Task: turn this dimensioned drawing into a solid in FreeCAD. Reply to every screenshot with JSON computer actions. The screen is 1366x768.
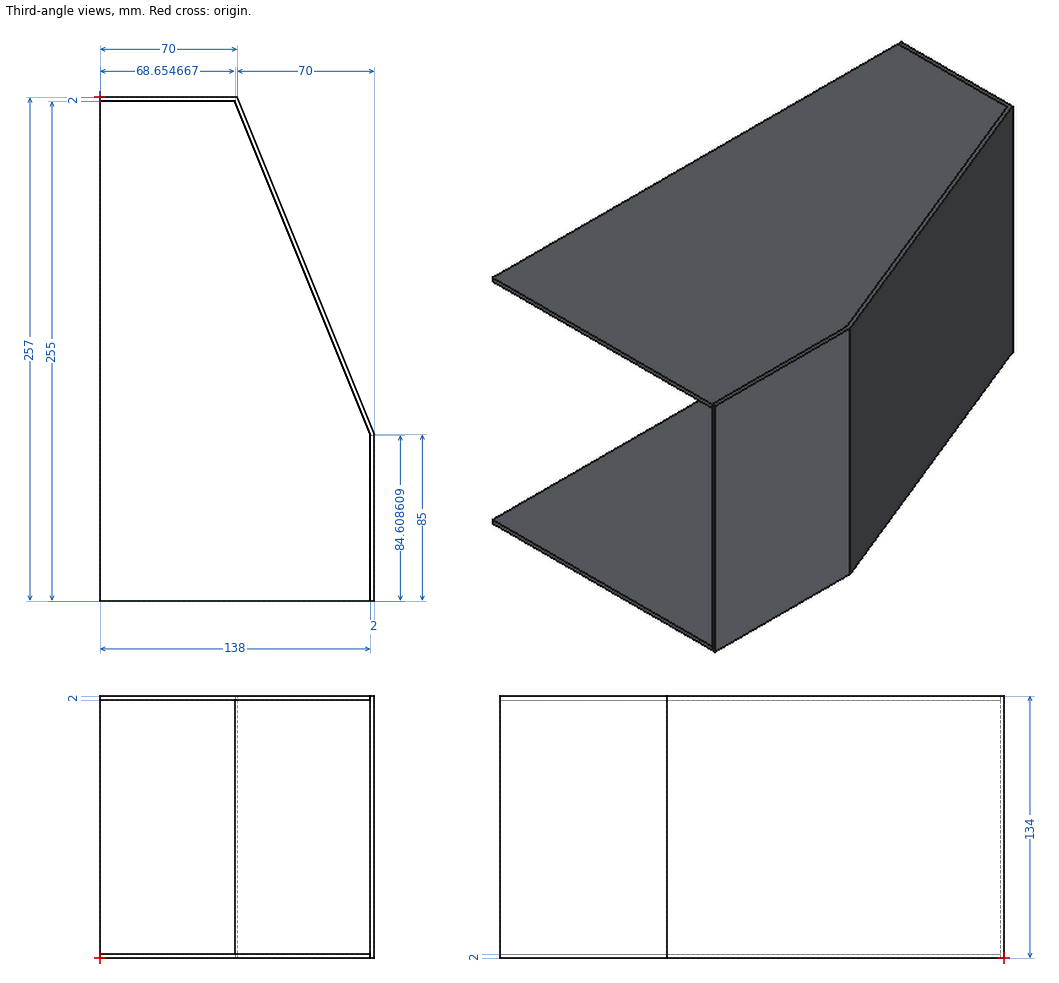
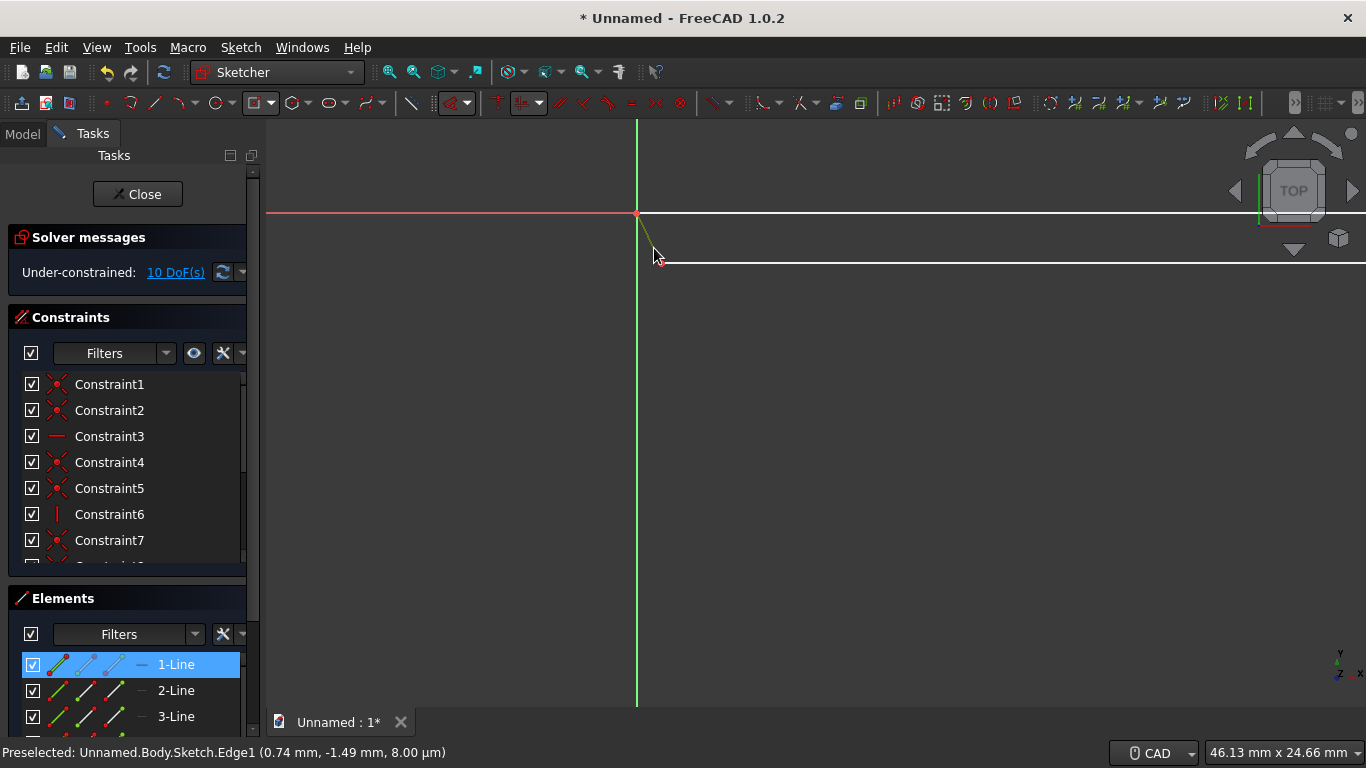
{"action": "key", "text": "v"}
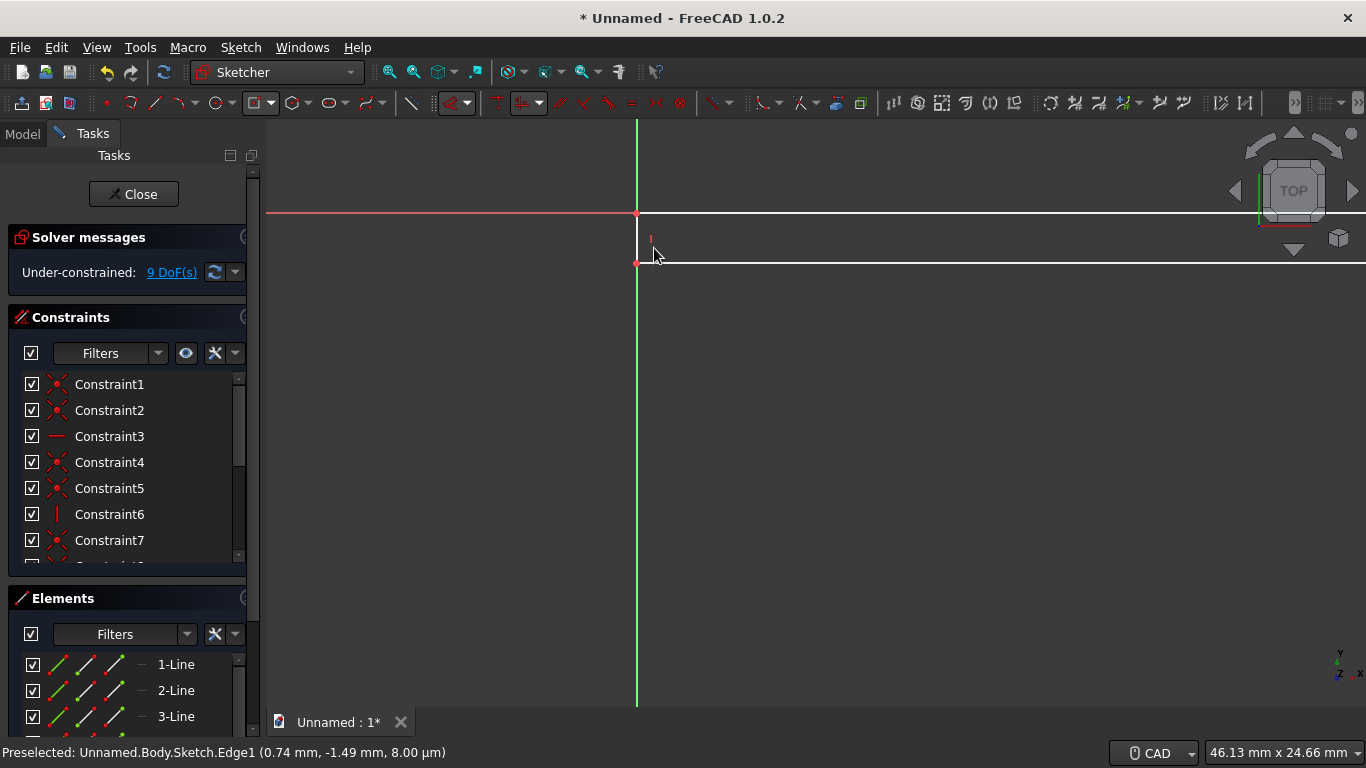
{"action": "scroll", "coordinate": [647, 228], "scroll_direction": "down", "scroll_amount": 14}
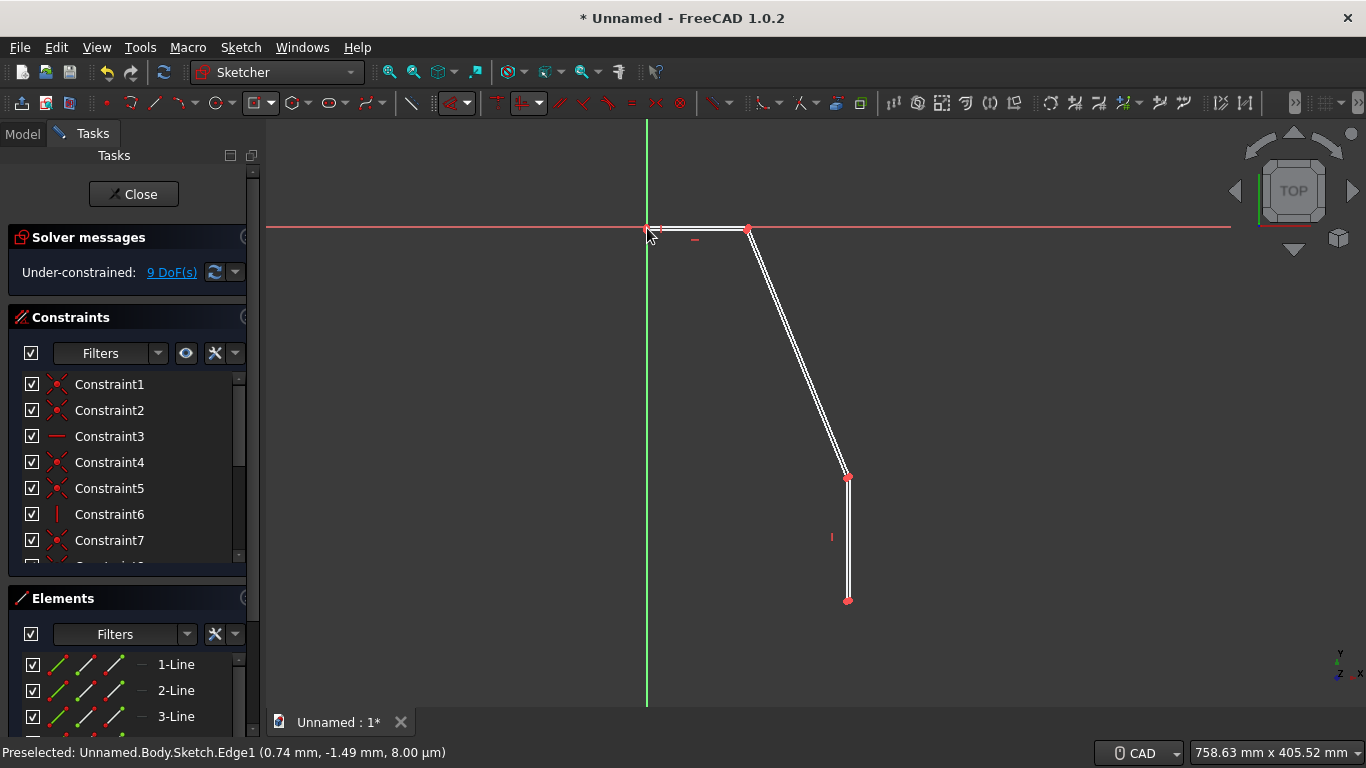
{"action": "scroll", "coordinate": [848, 601], "scroll_direction": "up", "scroll_amount": 14}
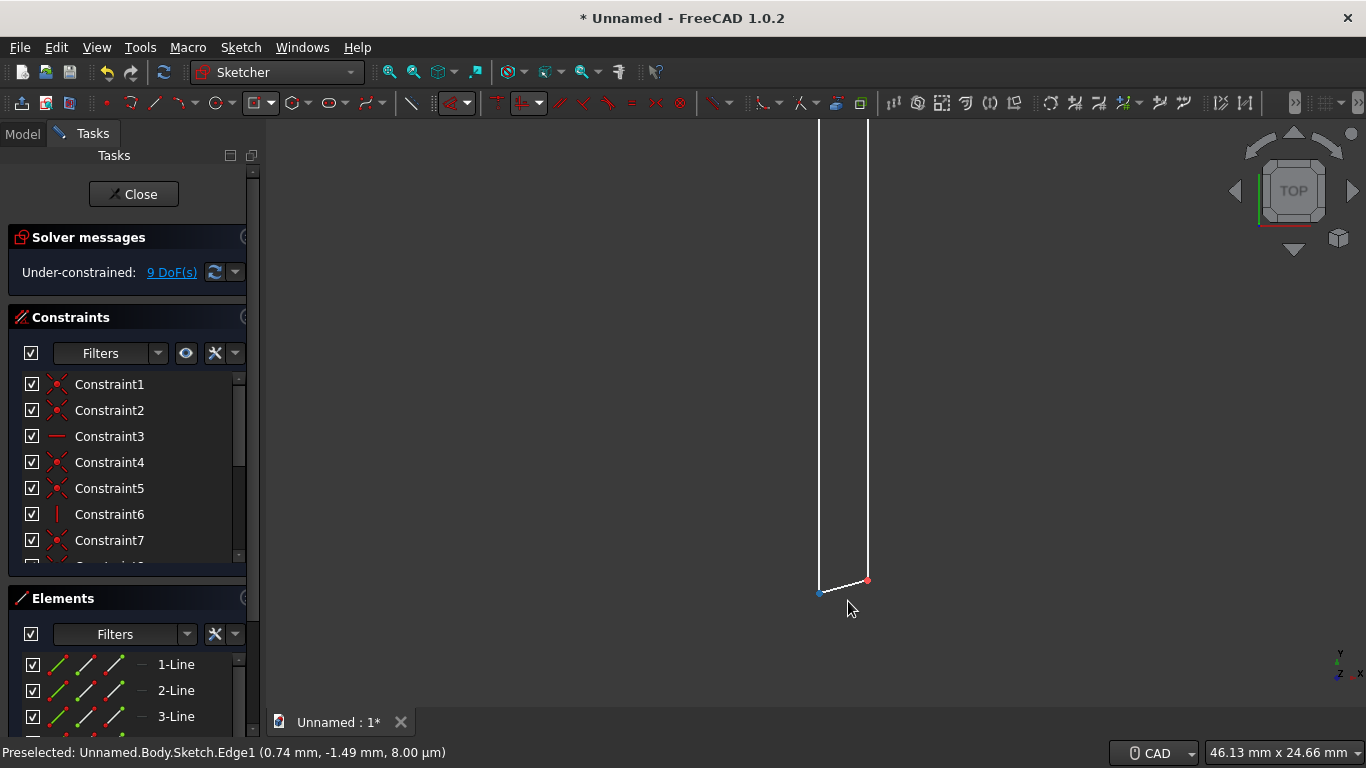
{"action": "left_click", "coordinate": [834, 589]}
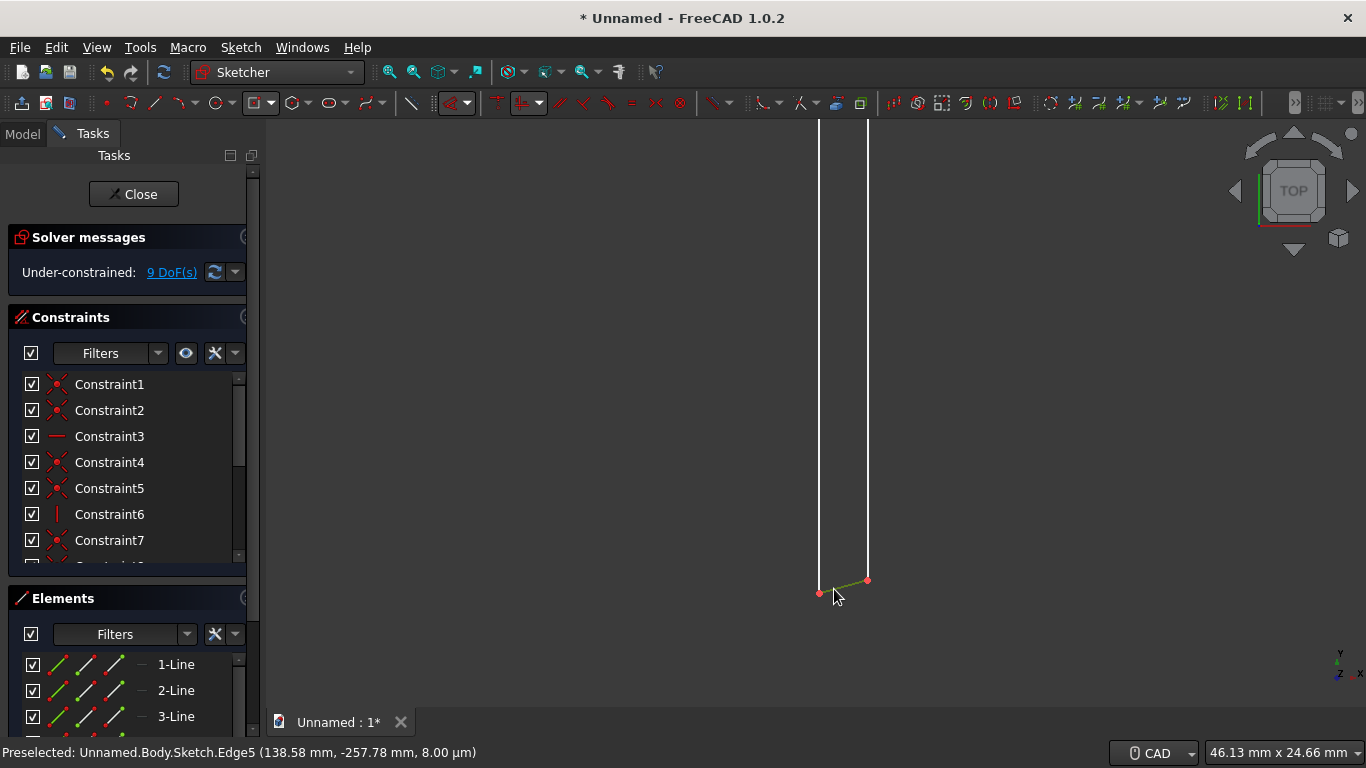
{"action": "key", "text": "h"}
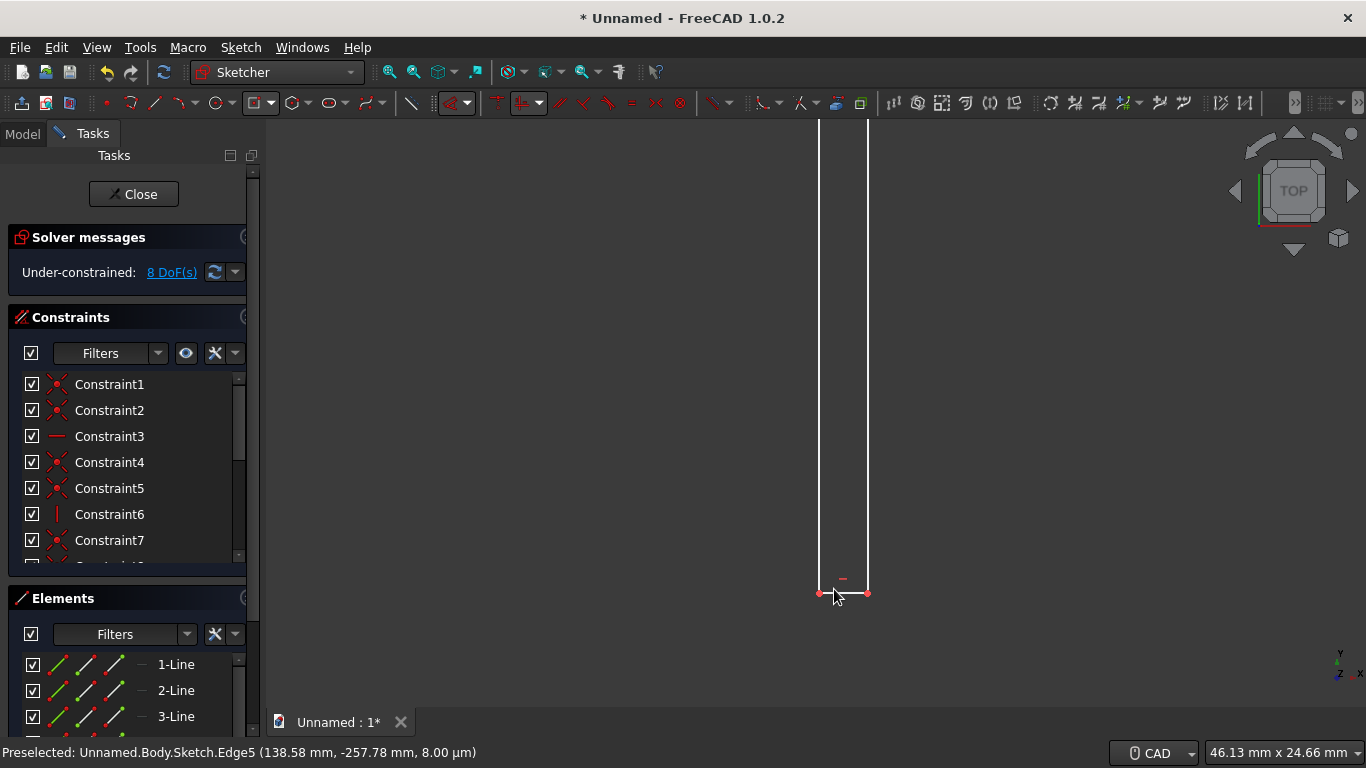
{"action": "key", "text": "d"}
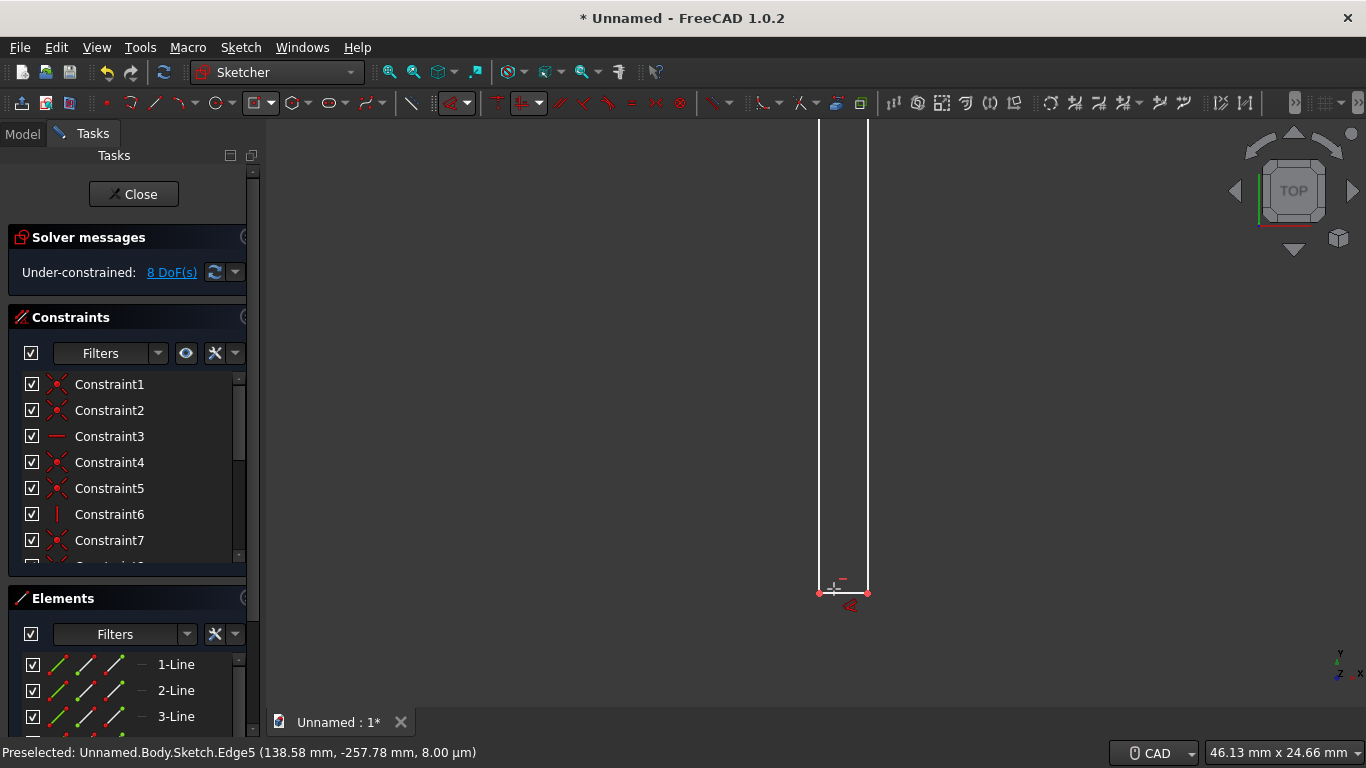
{"action": "scroll", "coordinate": [848, 601], "scroll_direction": "down", "scroll_amount": 14}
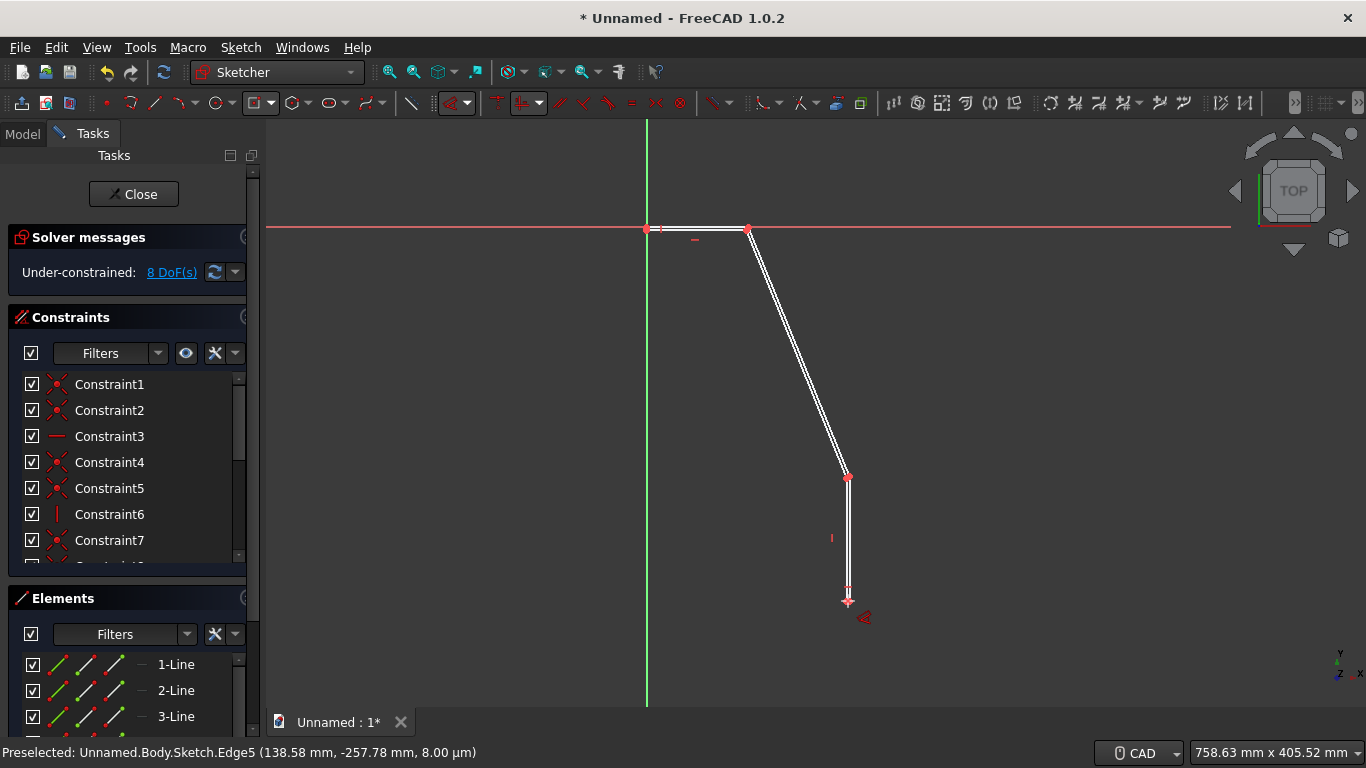
{"action": "scroll", "coordinate": [647, 228], "scroll_direction": "up", "scroll_amount": 14}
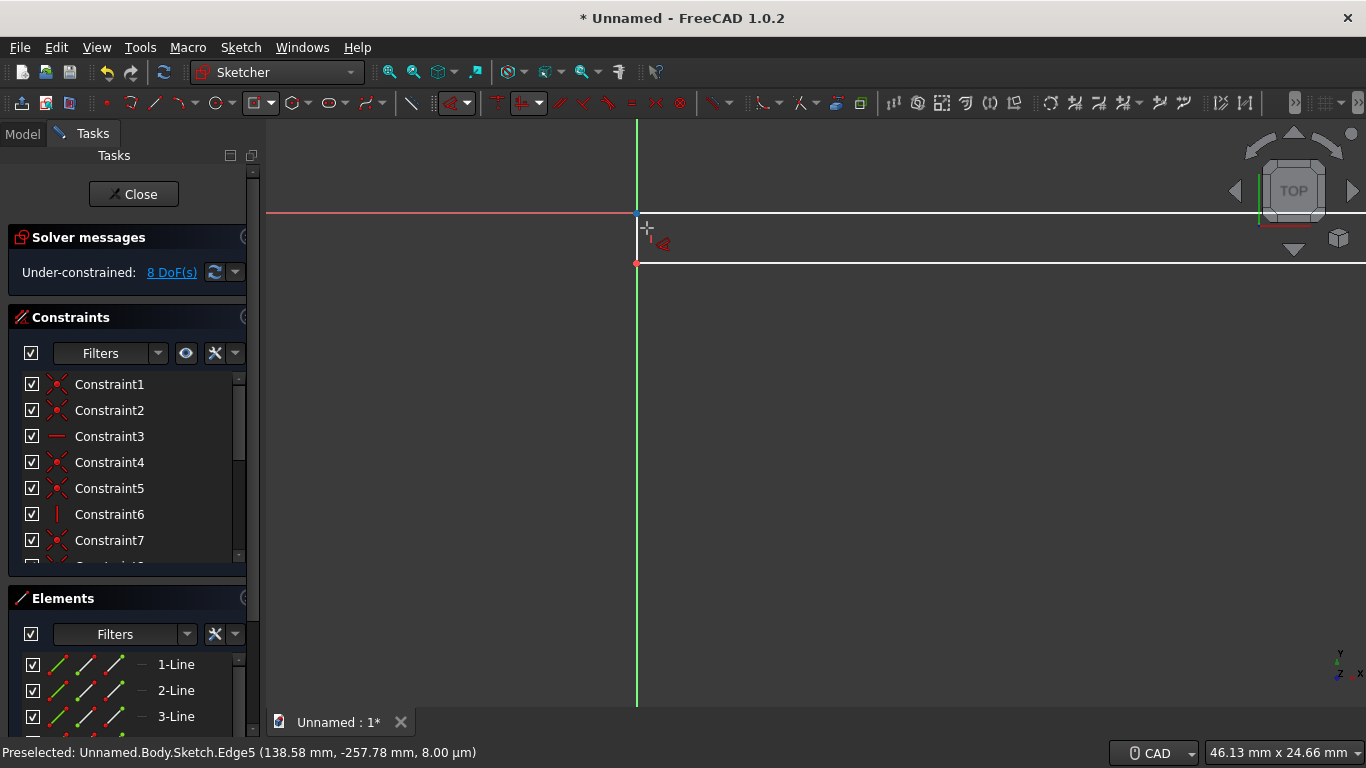
{"action": "left_click", "coordinate": [637, 228]}
{"action": "left_click", "coordinate": [603, 238]}